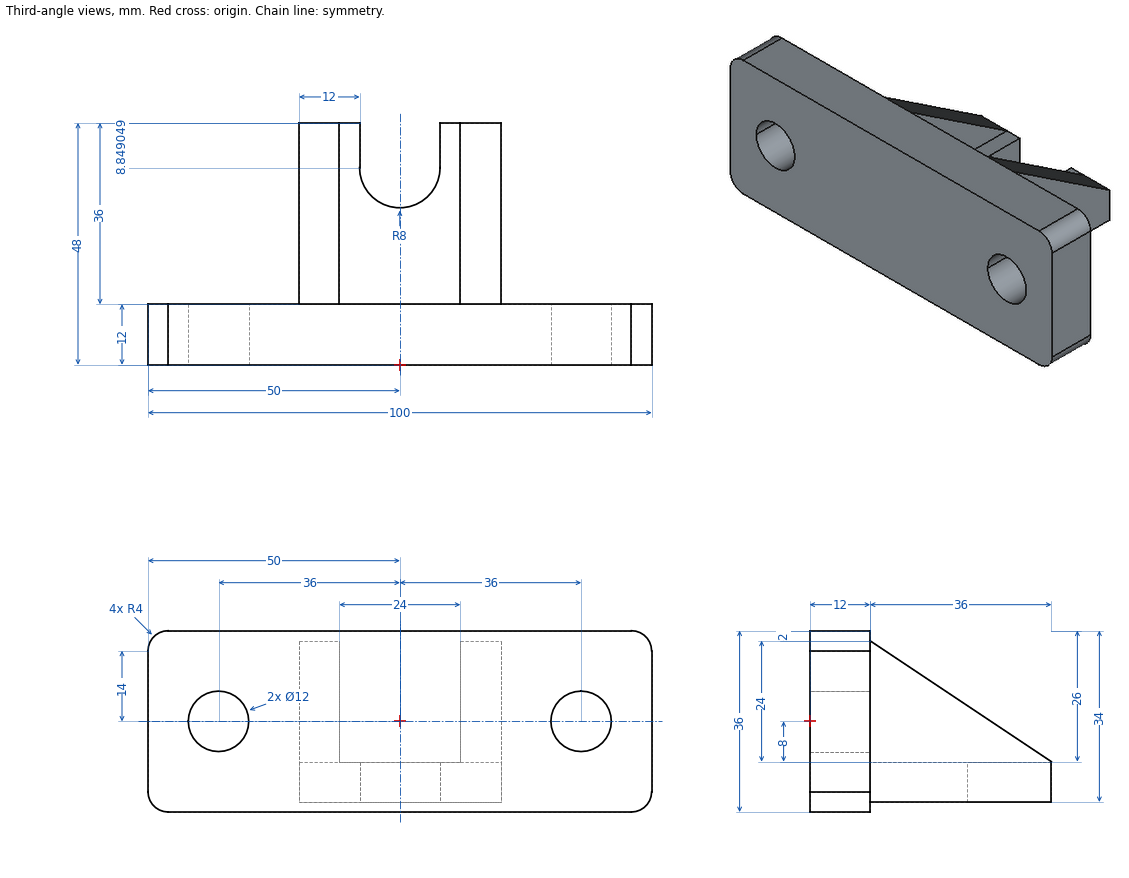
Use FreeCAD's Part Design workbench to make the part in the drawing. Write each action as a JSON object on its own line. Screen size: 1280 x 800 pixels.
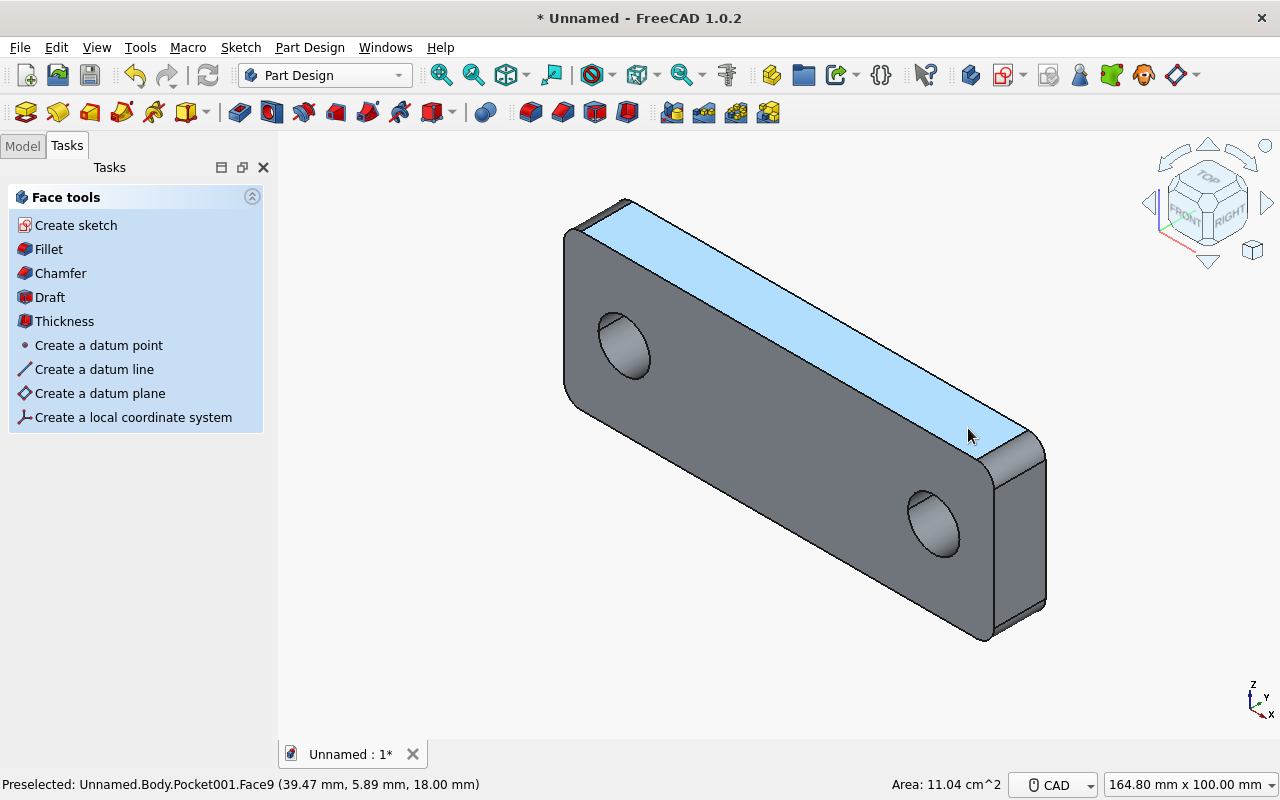
{"action": "left_click", "coordinate": [1004, 76]}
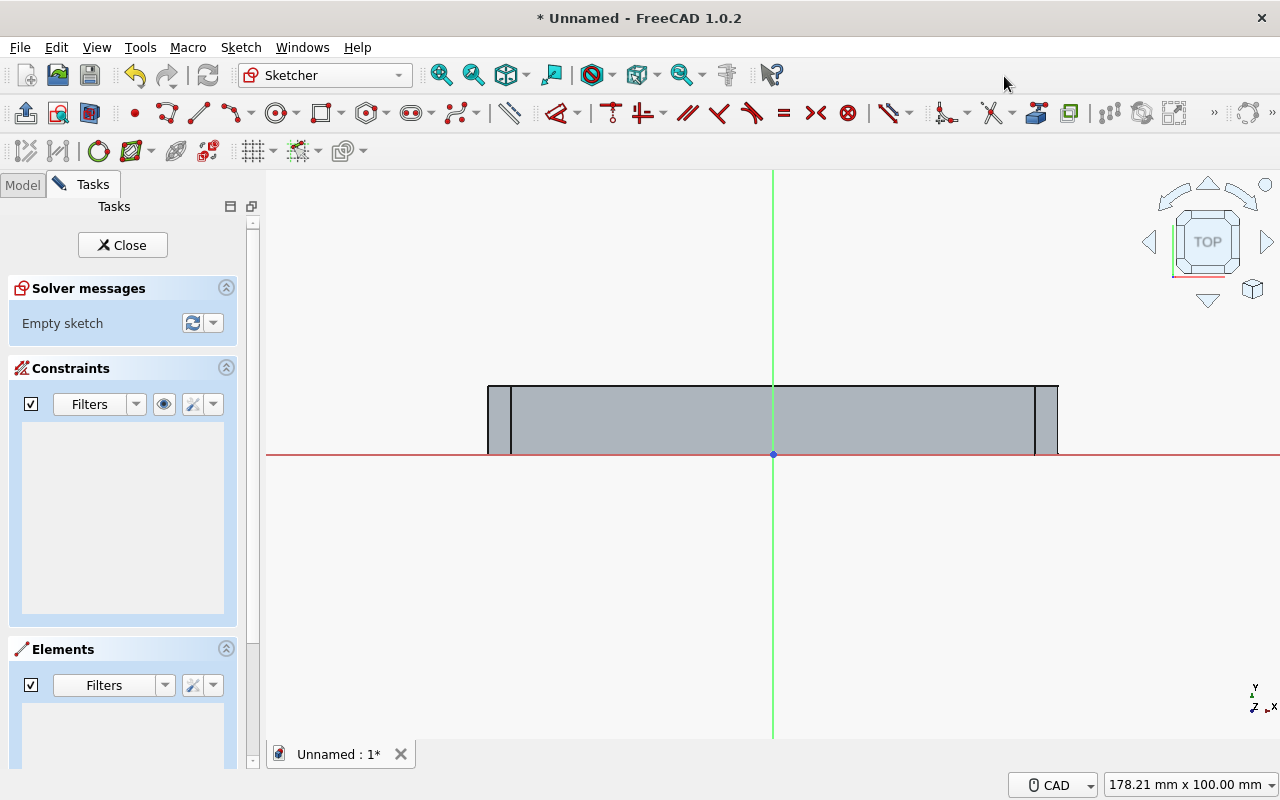
{"action": "scroll", "coordinate": [395, 711], "scroll_direction": "down", "scroll_amount": 1}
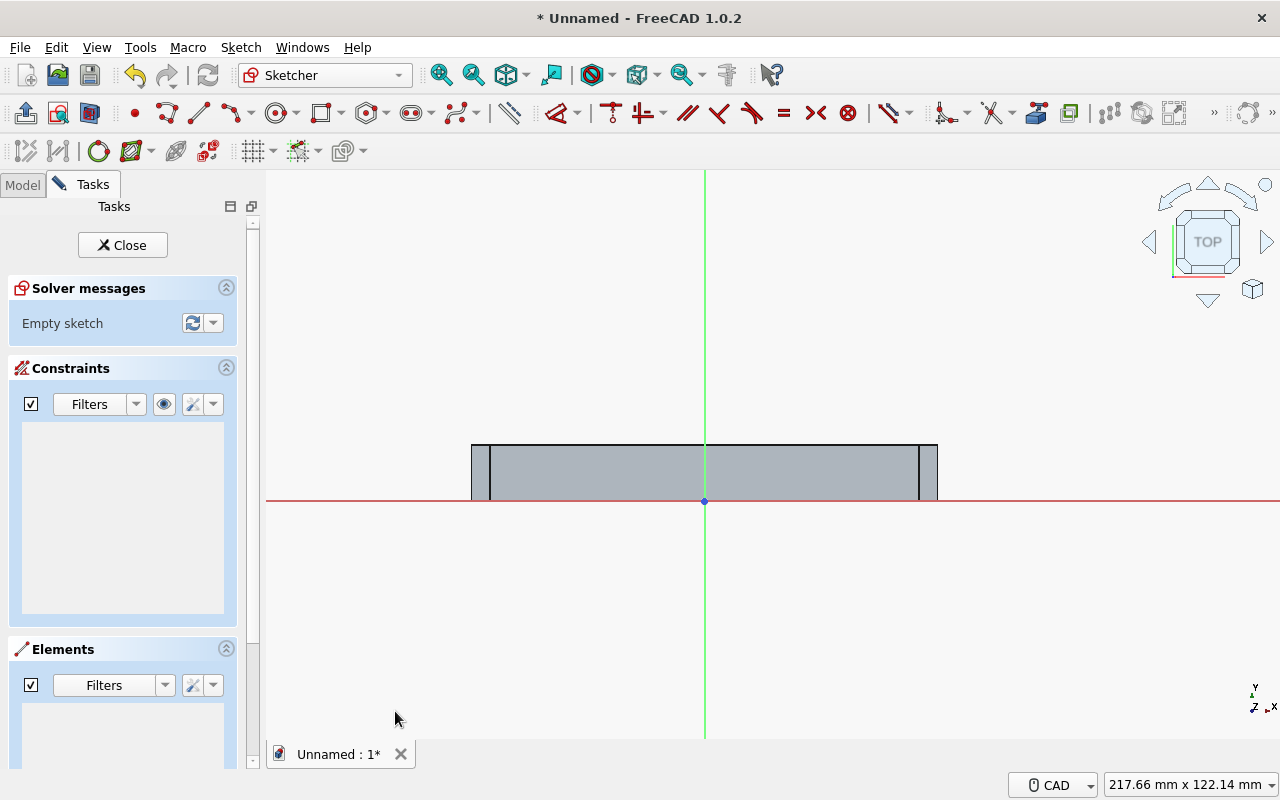
{"action": "scroll", "coordinate": [705, 257], "scroll_direction": "up", "scroll_amount": 2}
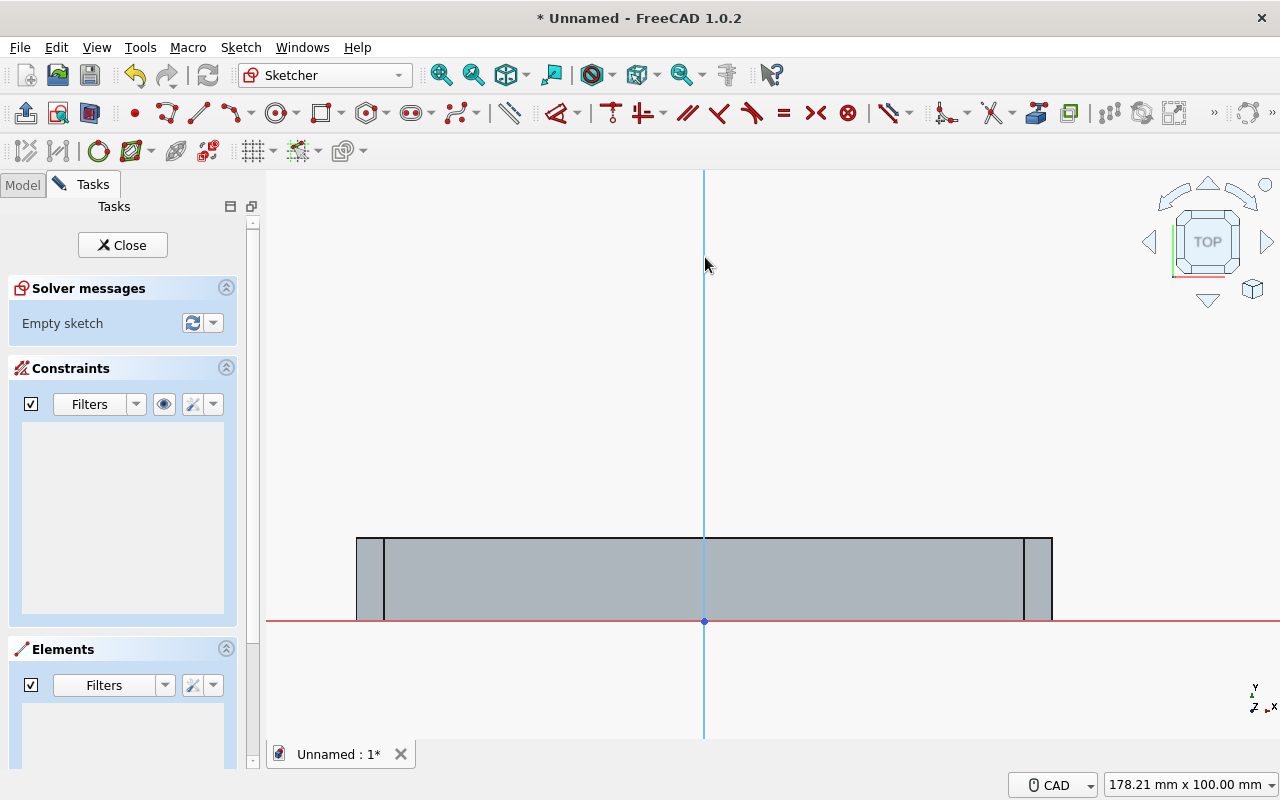
{"action": "left_click", "coordinate": [168, 114]}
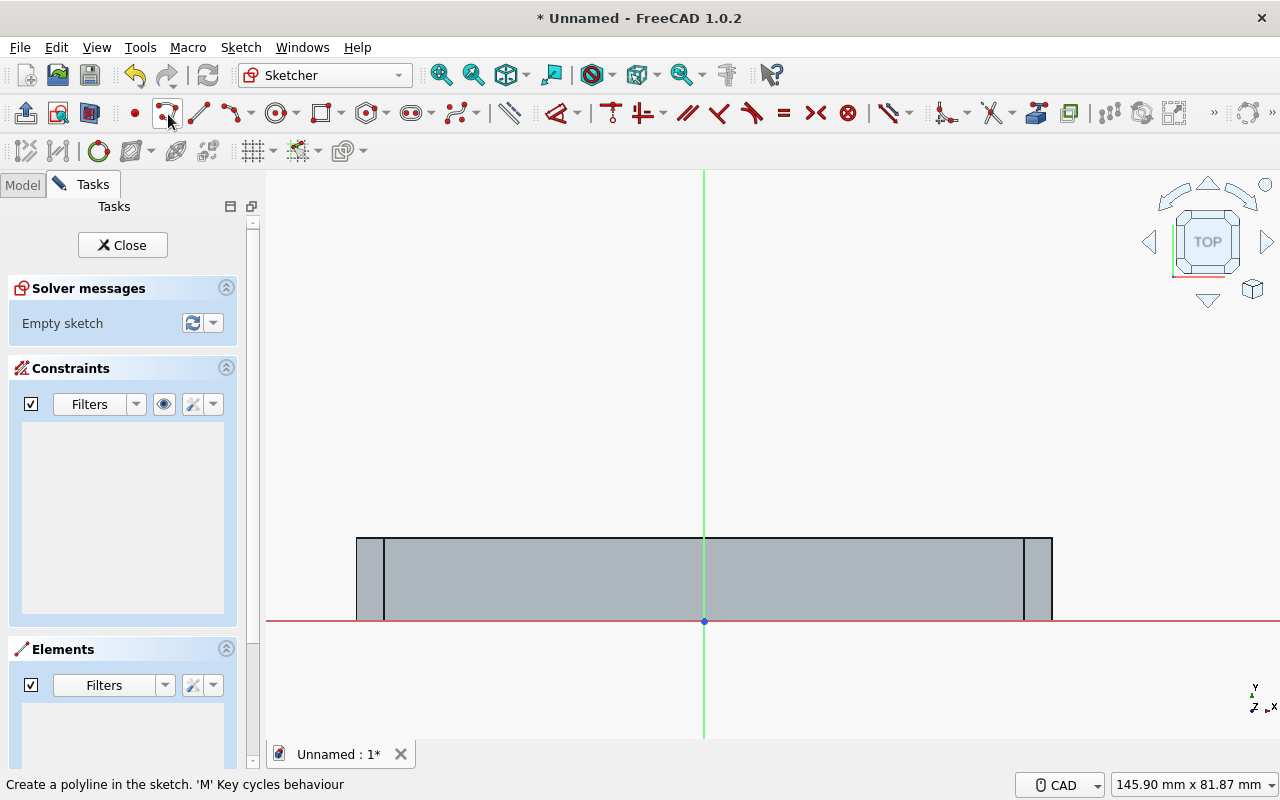
{"action": "left_click", "coordinate": [648, 349]}
{"action": "left_click", "coordinate": [648, 288]}
{"action": "left_click", "coordinate": [565, 288]}
{"action": "left_click", "coordinate": [565, 538]}
{"action": "left_click", "coordinate": [843, 538]}
{"action": "left_click", "coordinate": [843, 288]}
{"action": "left_click", "coordinate": [760, 288]}
{"action": "left_click", "coordinate": [760, 349]}
{"action": "right_click", "coordinate": [760, 349]}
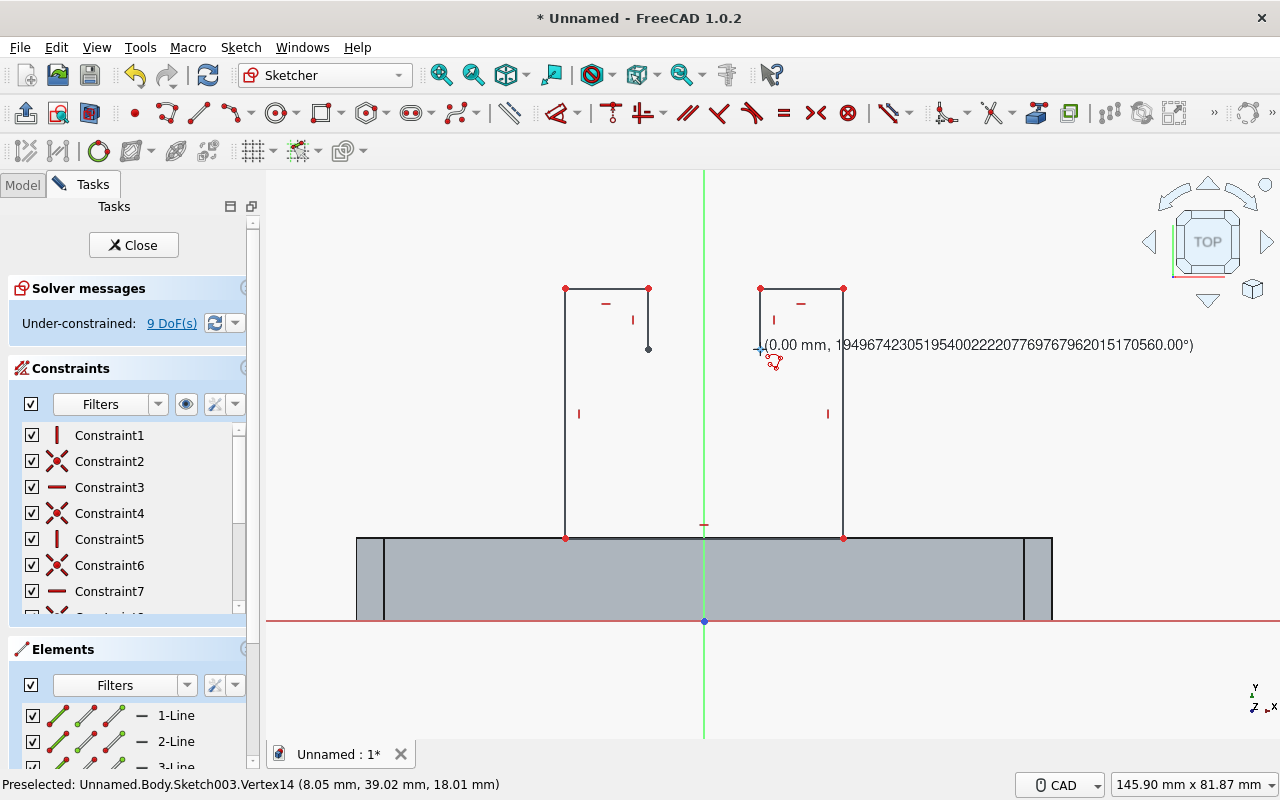
{"action": "left_click", "coordinate": [232, 114]}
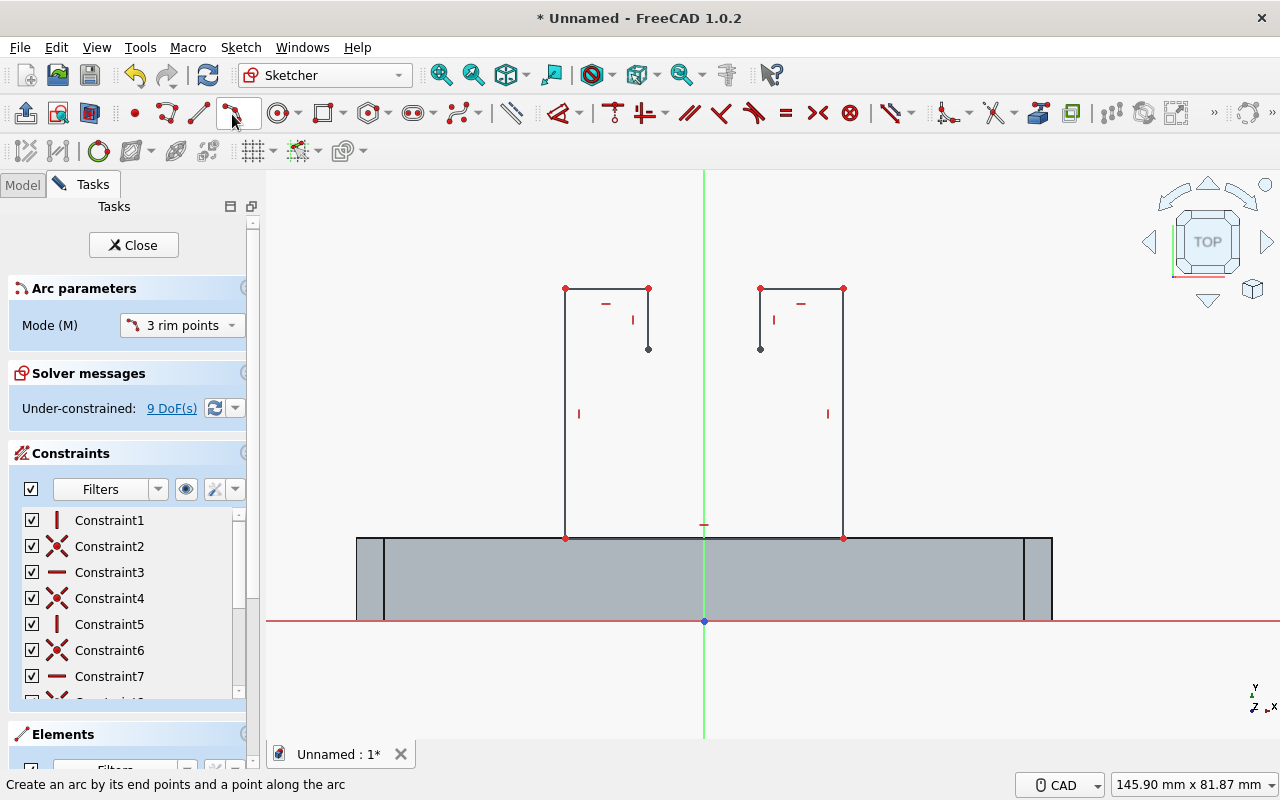
{"action": "left_click", "coordinate": [760, 350]}
{"action": "left_click", "coordinate": [648, 350]}
{"action": "left_click", "coordinate": [687, 402]}
{"action": "key", "text": "Escape"}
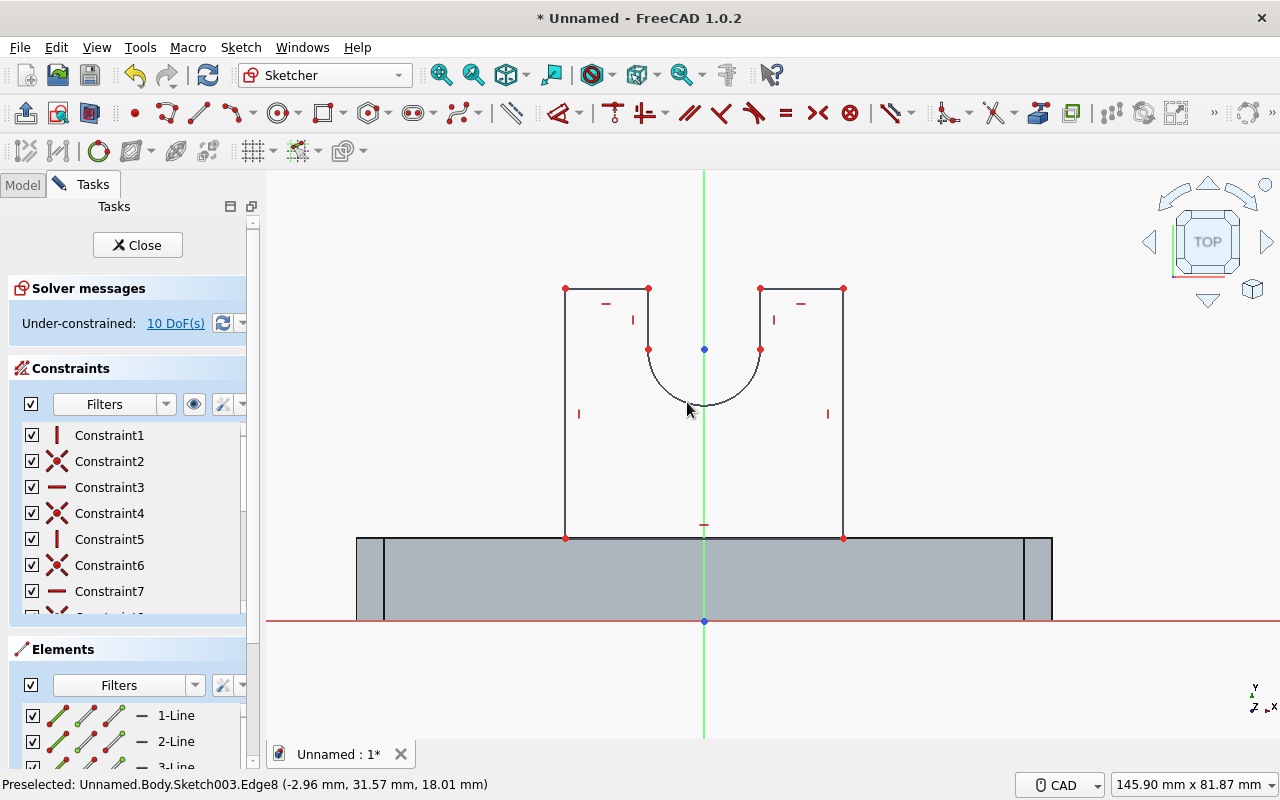
{"action": "left_click", "coordinate": [648, 332]}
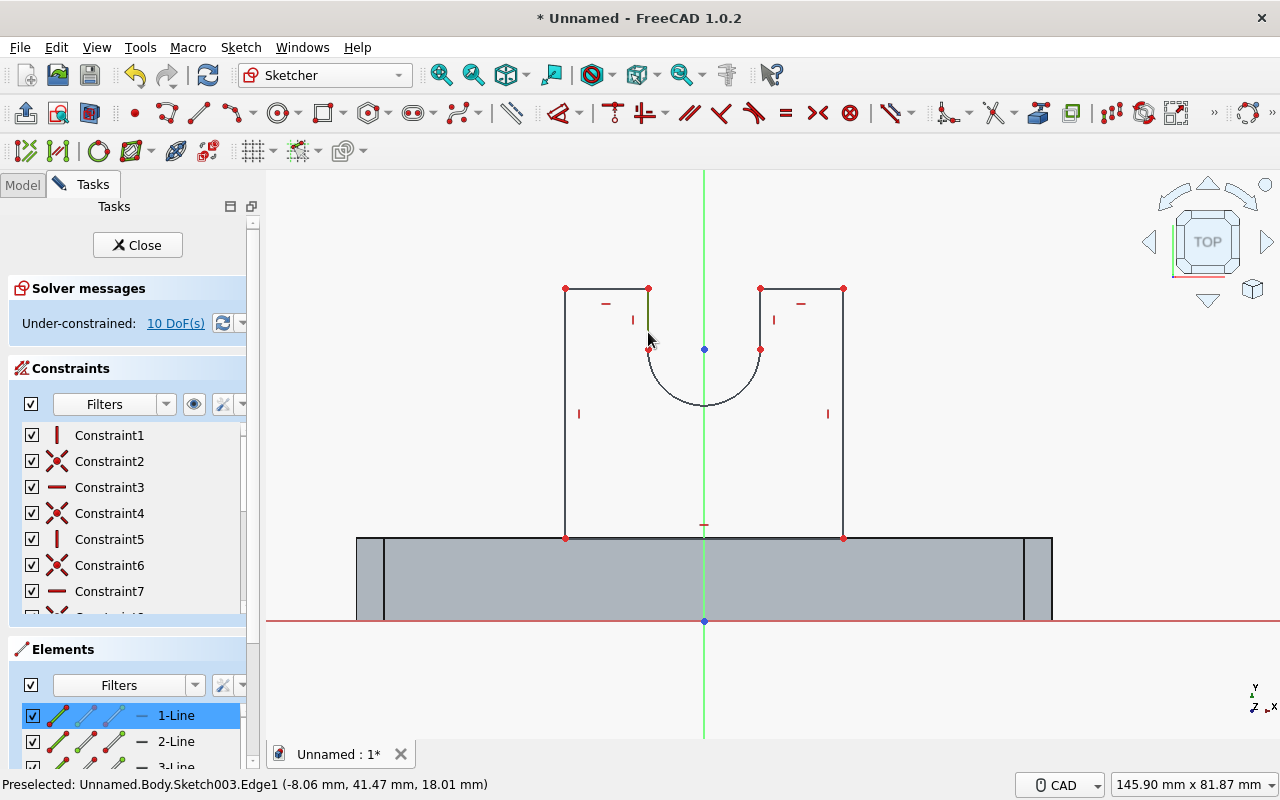
{"action": "left_click", "coordinate": [671, 395]}